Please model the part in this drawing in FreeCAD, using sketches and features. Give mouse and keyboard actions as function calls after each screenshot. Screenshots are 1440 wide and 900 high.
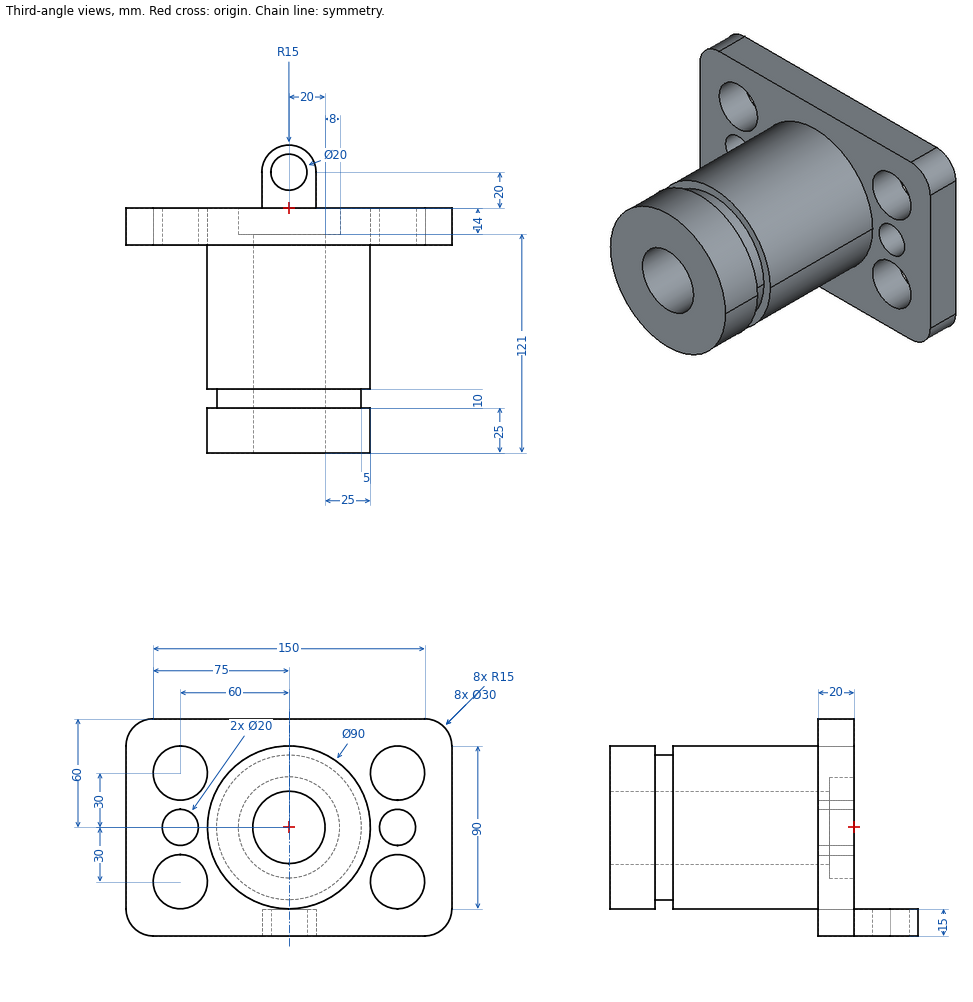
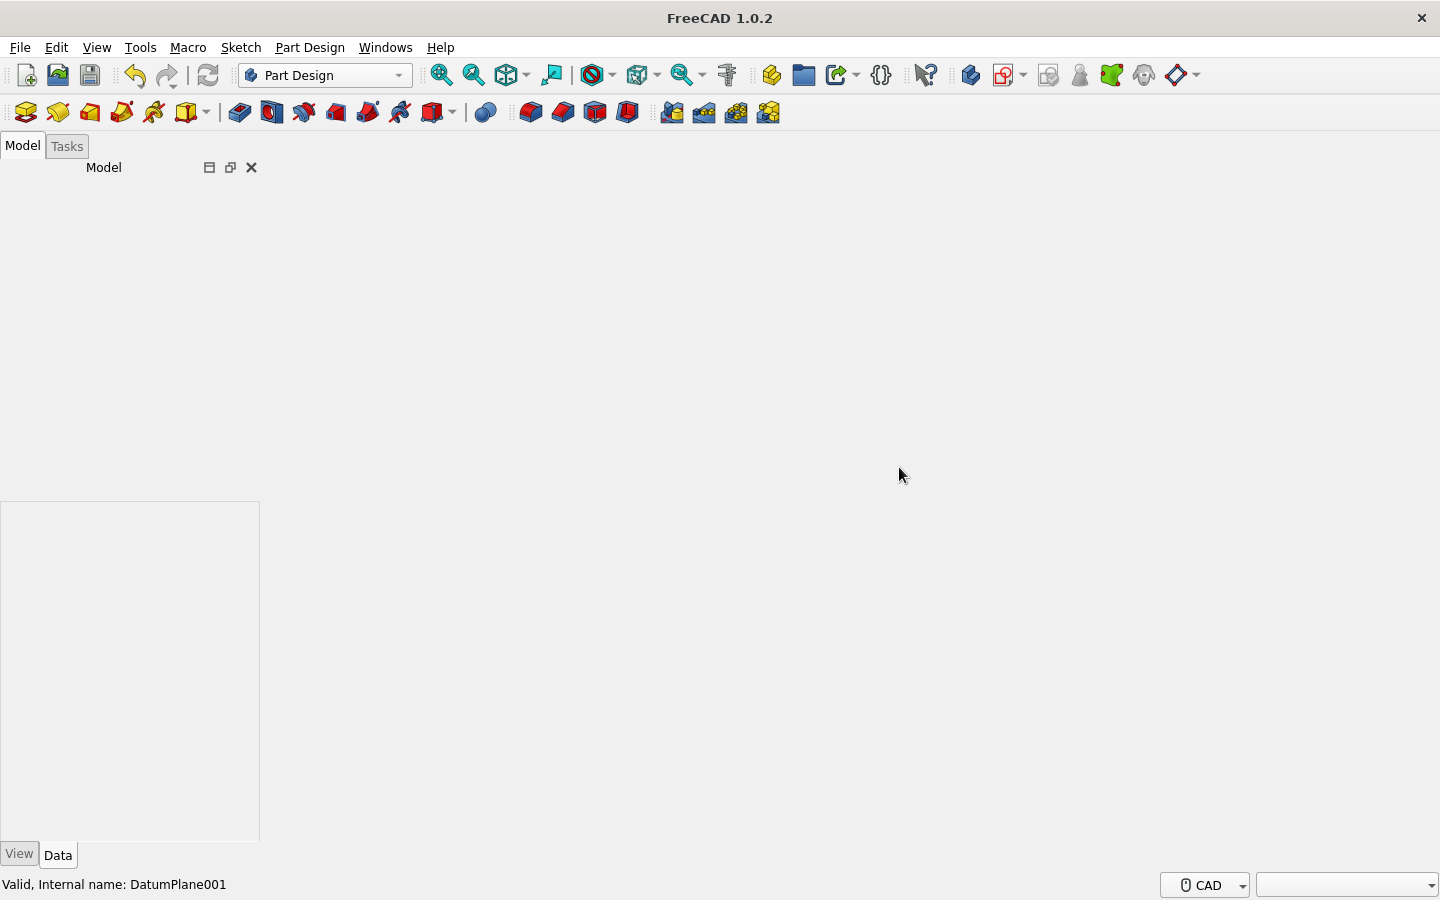
key(ctrl+n)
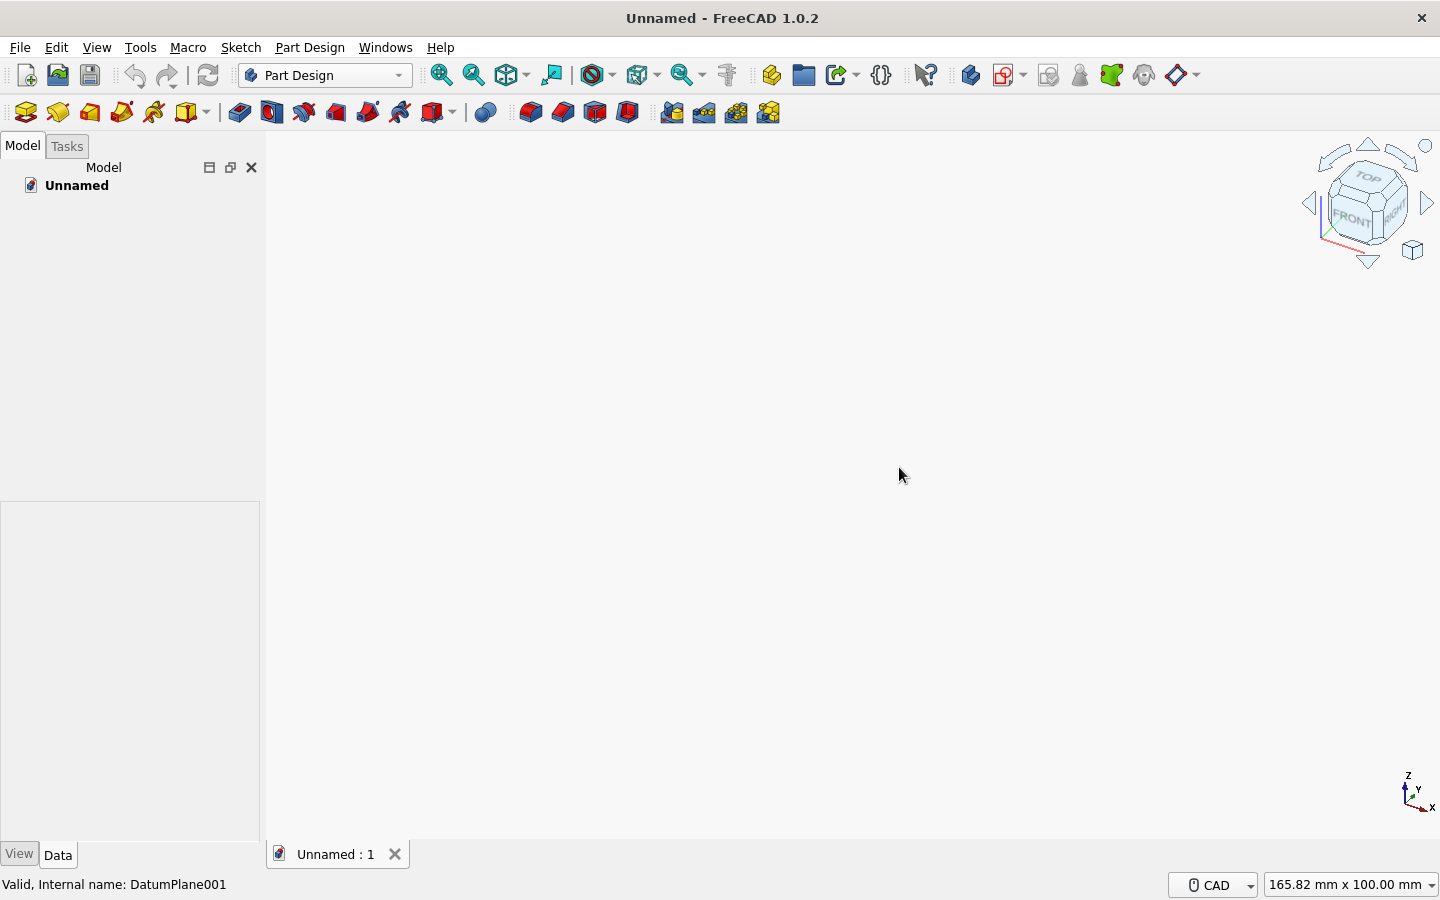
click(1004, 76)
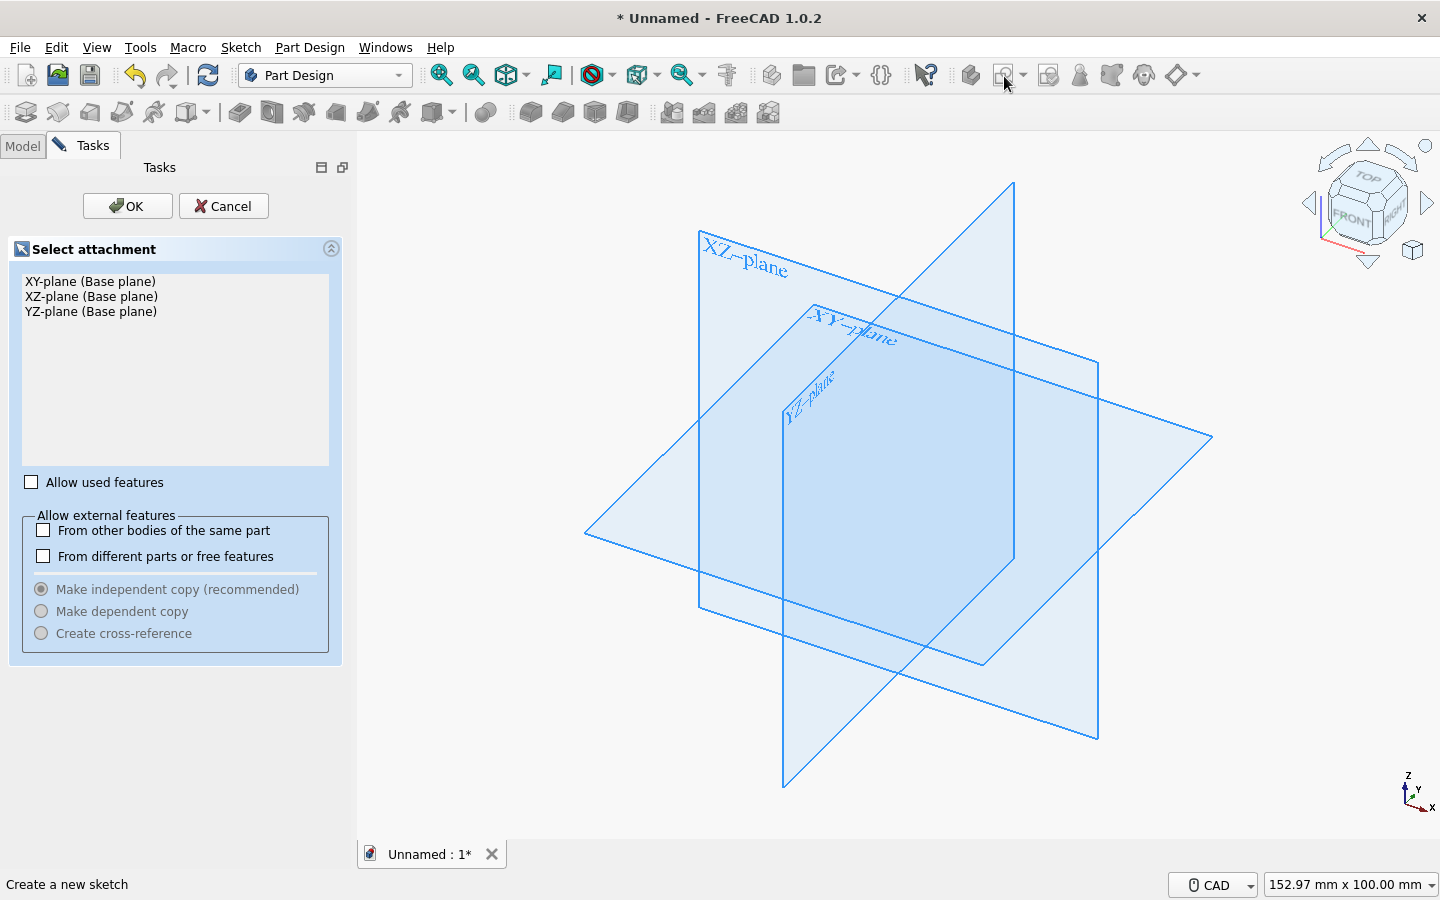
click(82, 282)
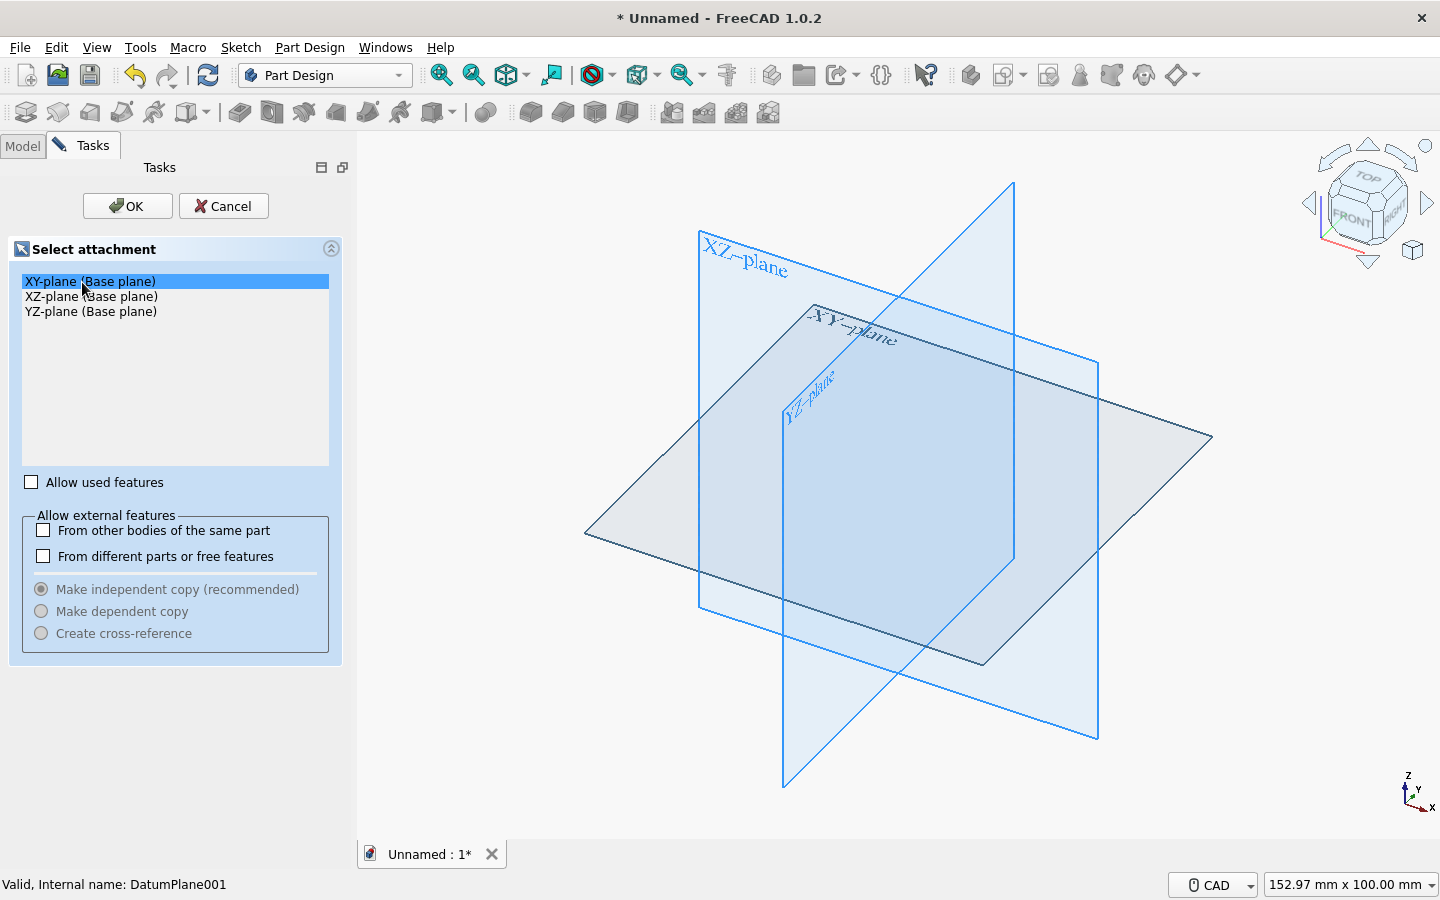
click(128, 206)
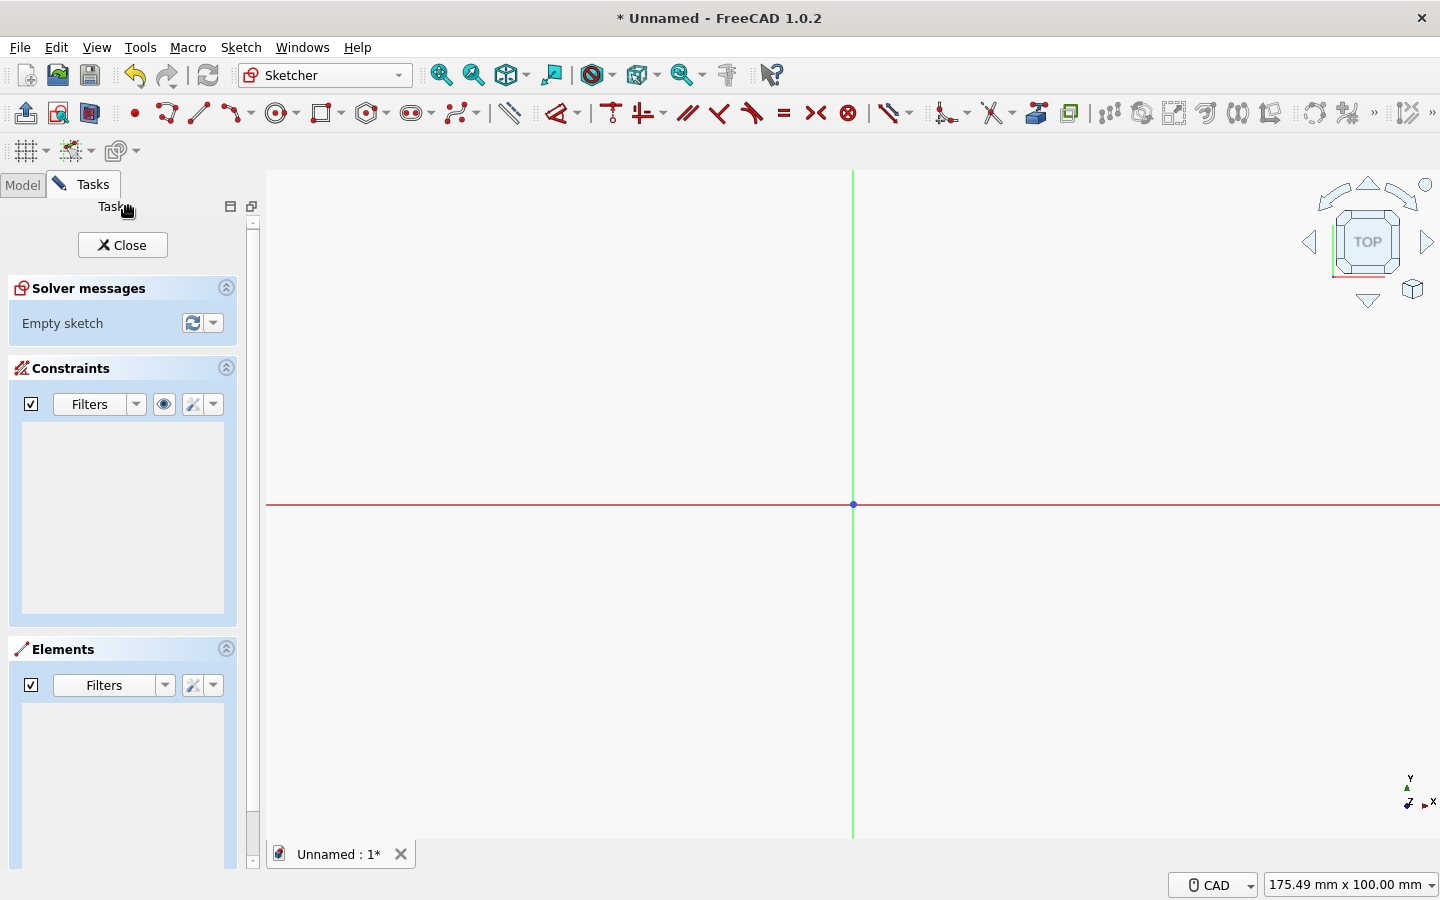
scroll(606, 198, down, 4)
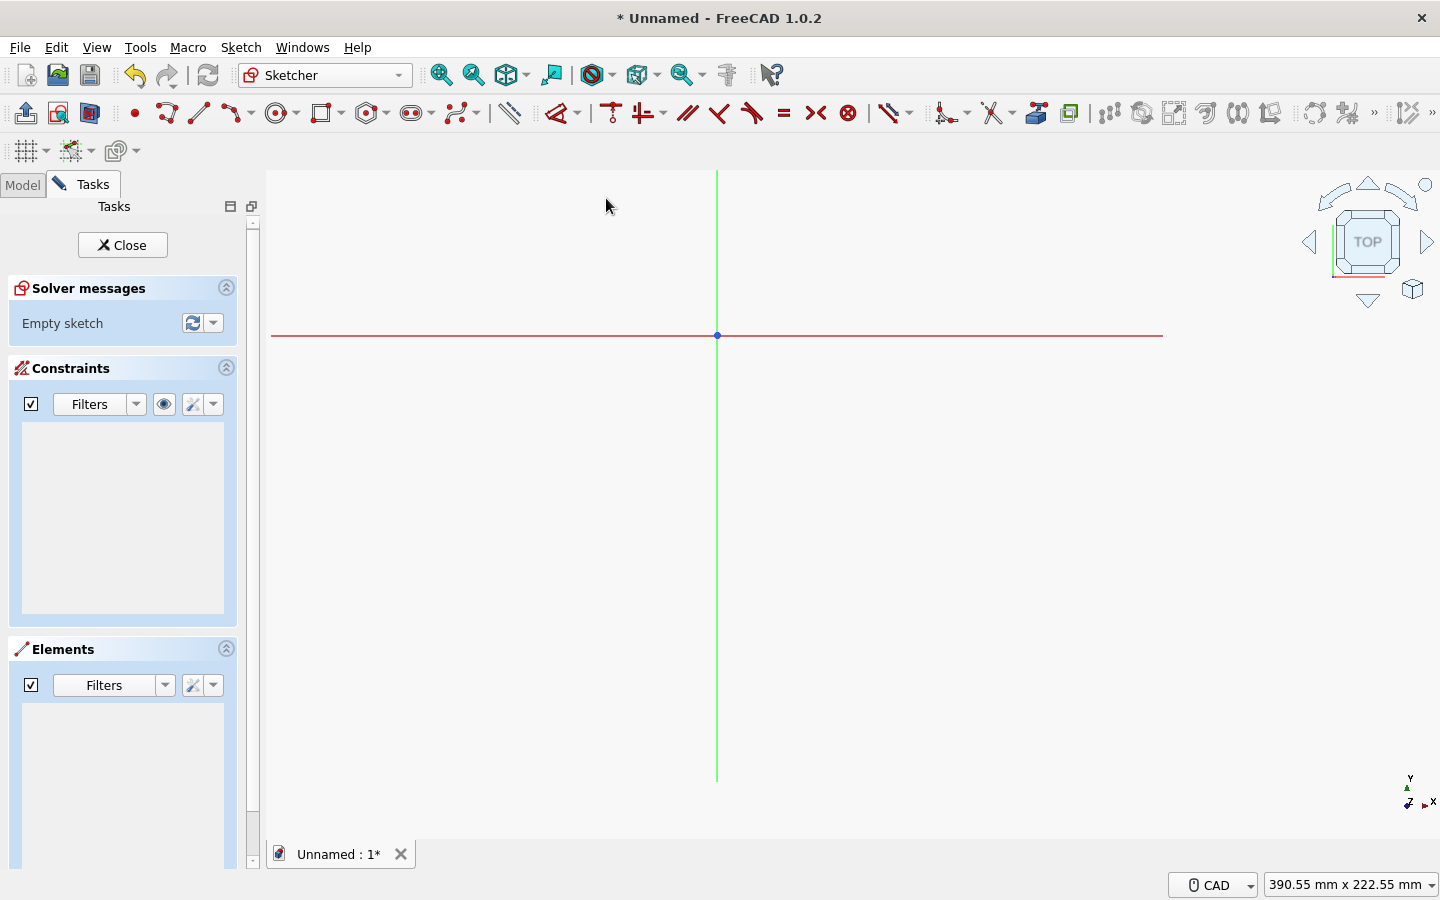
click(168, 114)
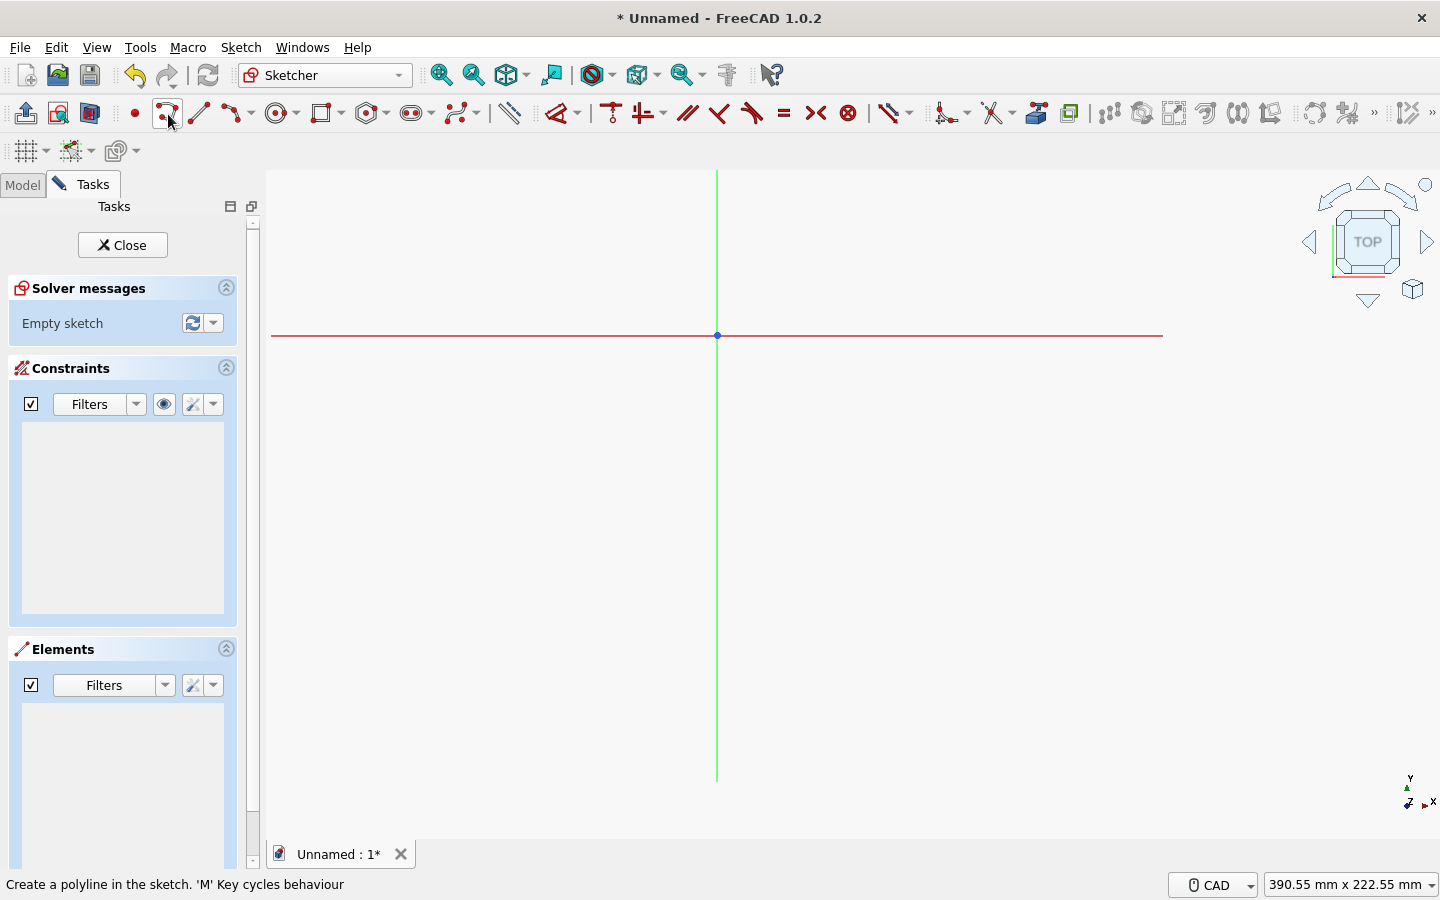
click(777, 378)
click(777, 742)
click(852, 742)
click(852, 666)
click(837, 666)
click(837, 636)
click(852, 636)
click(852, 336)
click(801, 345)
click(801, 378)
click(777, 379)
key(Escape)
key(Escape)